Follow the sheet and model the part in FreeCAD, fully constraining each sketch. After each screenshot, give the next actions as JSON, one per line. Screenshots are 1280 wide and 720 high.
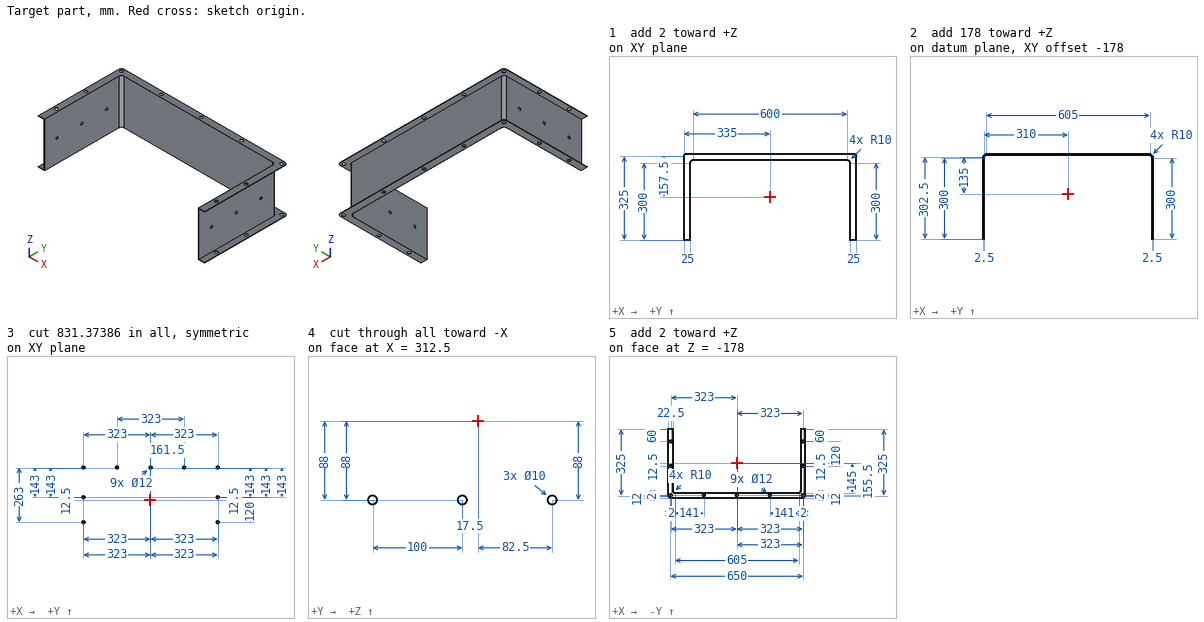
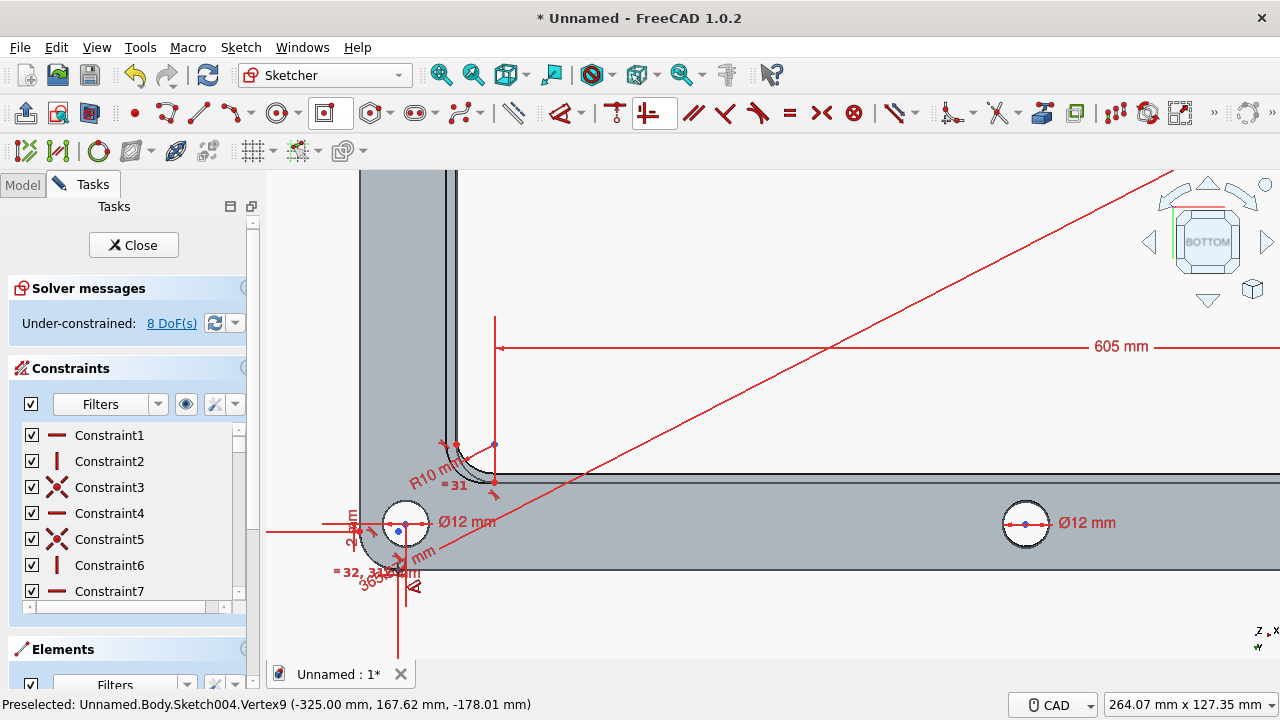
{"action": "left_click", "coordinate": [1026, 525]}
{"action": "left_click", "coordinate": [1060, 548]}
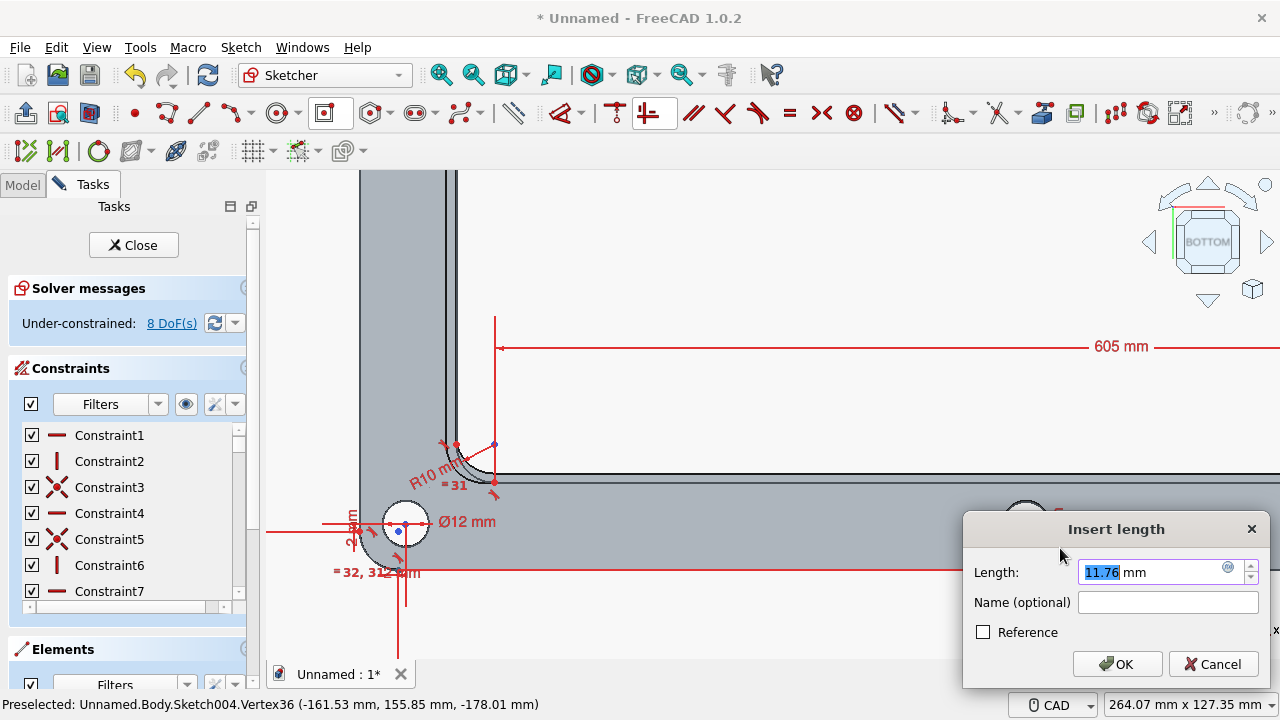
{"action": "type", "text": "12"}
{"action": "key", "text": "Return"}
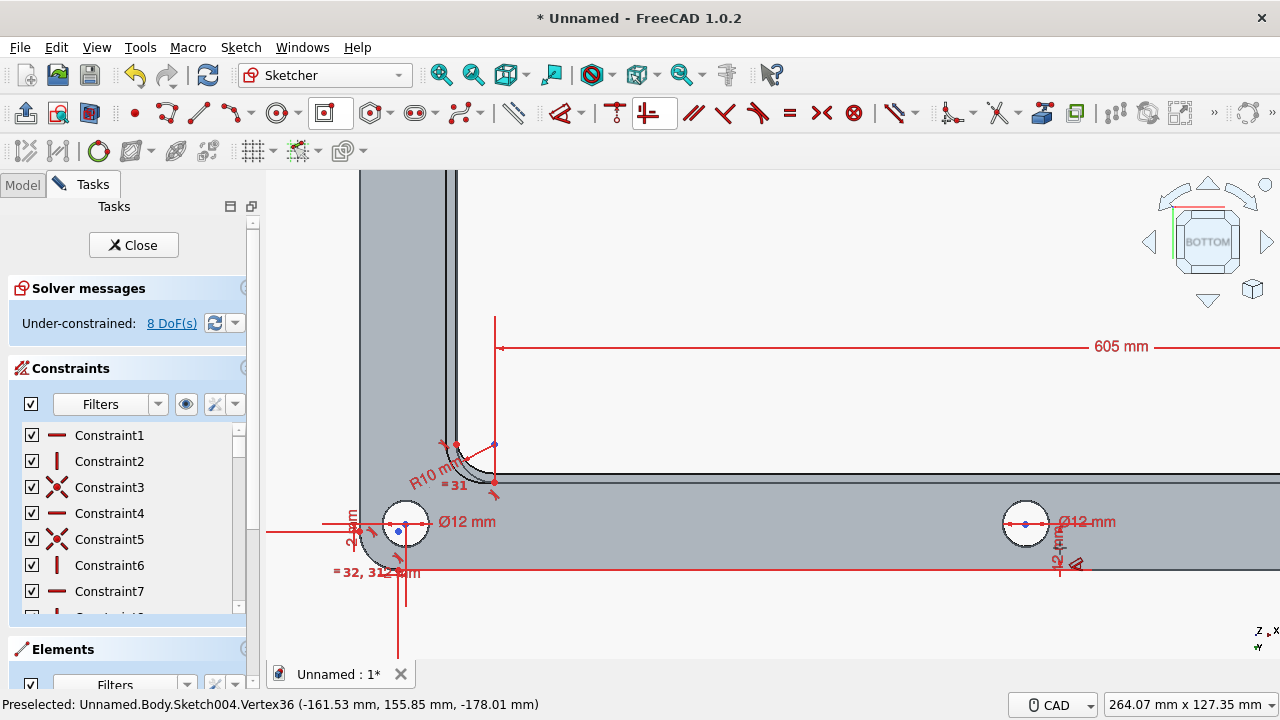
{"action": "scroll", "coordinate": [396, 574], "scroll_direction": "down", "scroll_amount": 7}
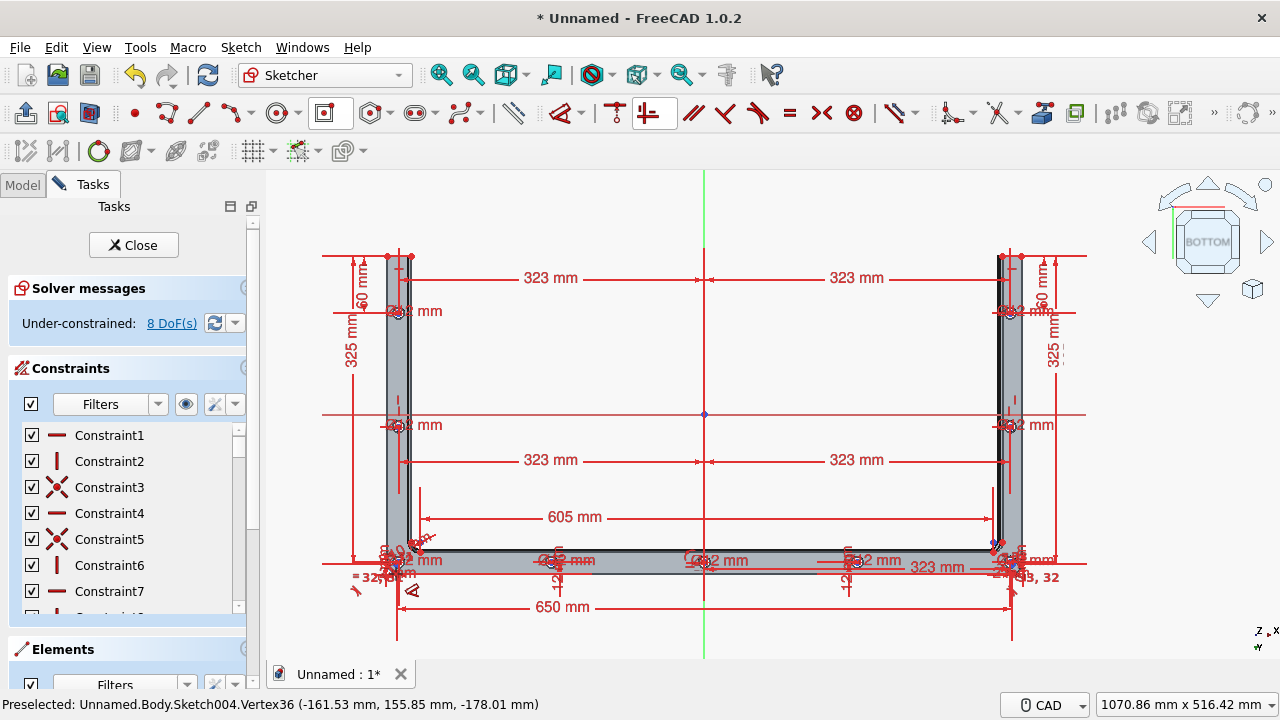
{"action": "scroll", "coordinate": [404, 256], "scroll_direction": "up", "scroll_amount": 4}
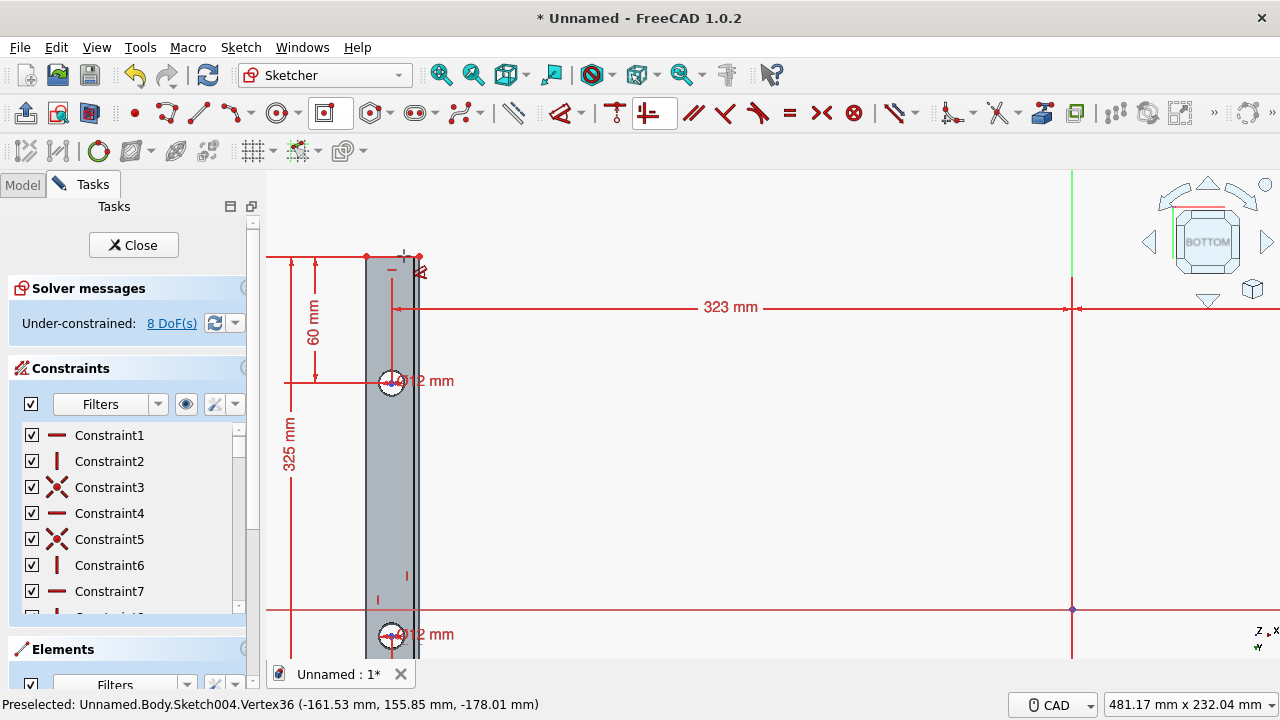
{"action": "left_click", "coordinate": [404, 257]}
{"action": "left_click", "coordinate": [393, 223]}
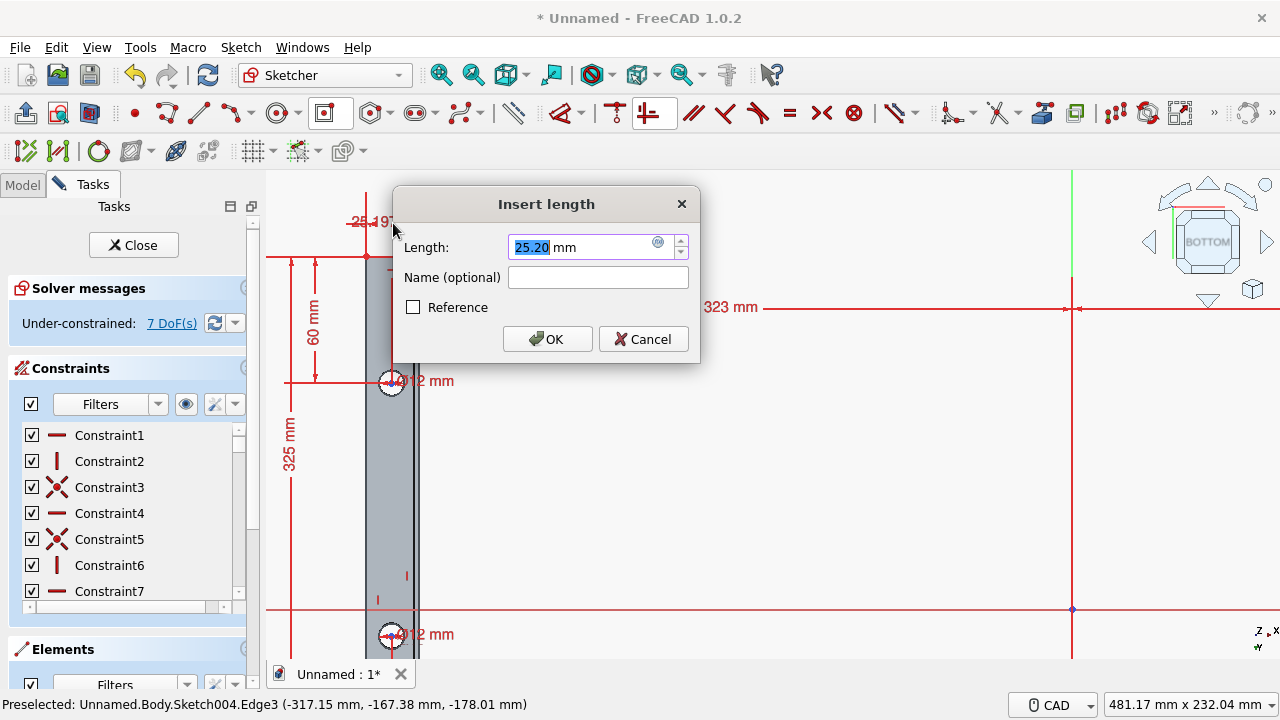
{"action": "type", "text": "22.5"}
{"action": "key", "text": "Return"}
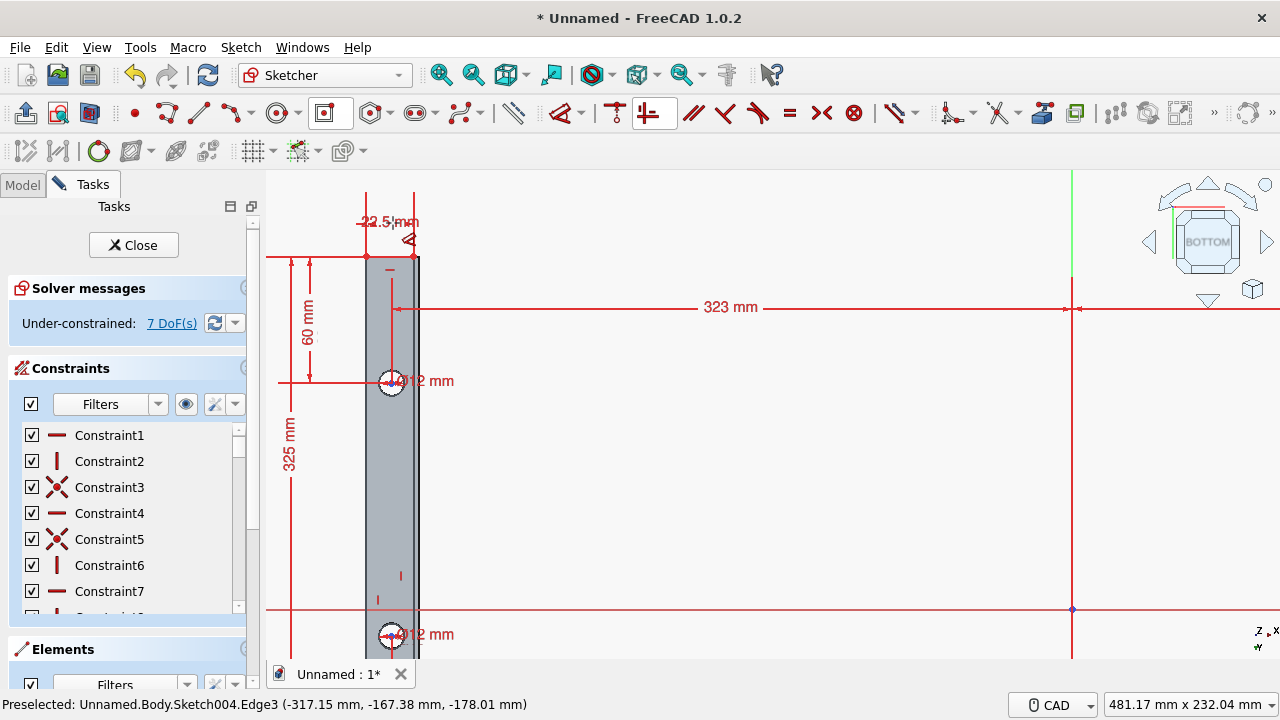
{"action": "scroll", "coordinate": [404, 255], "scroll_direction": "down", "scroll_amount": 4}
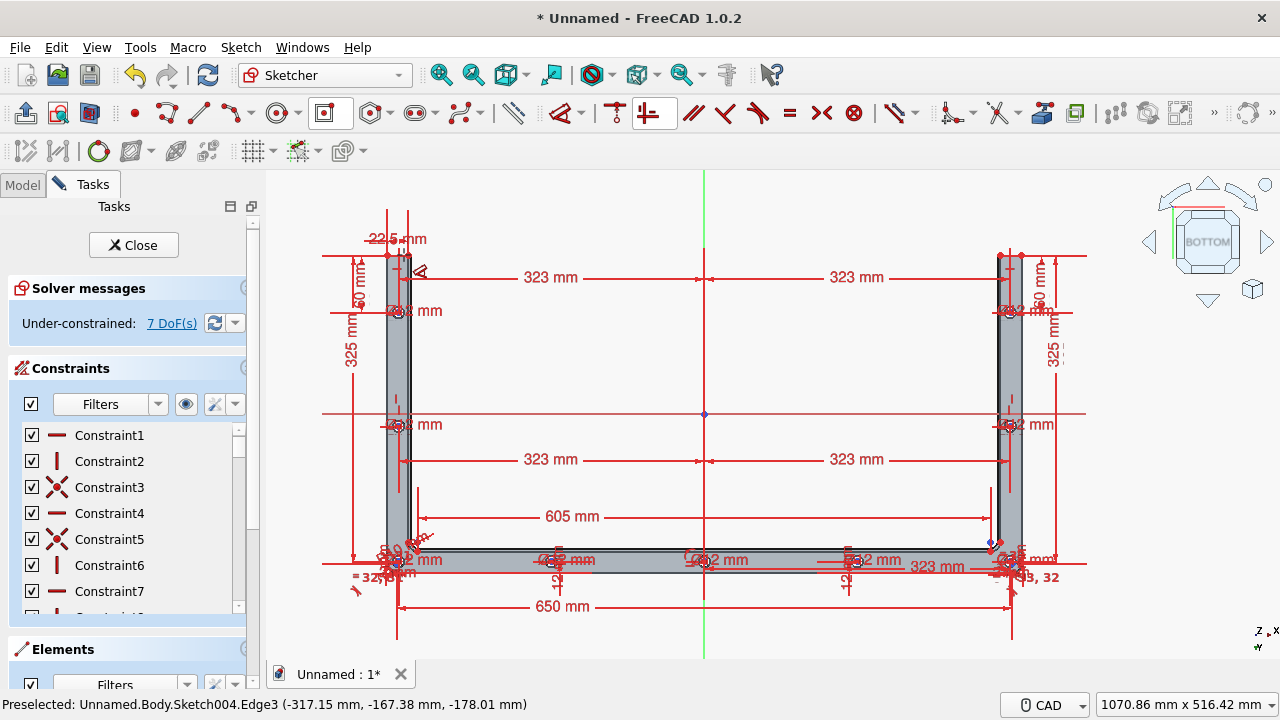
{"action": "scroll", "coordinate": [991, 552], "scroll_direction": "up", "scroll_amount": 2}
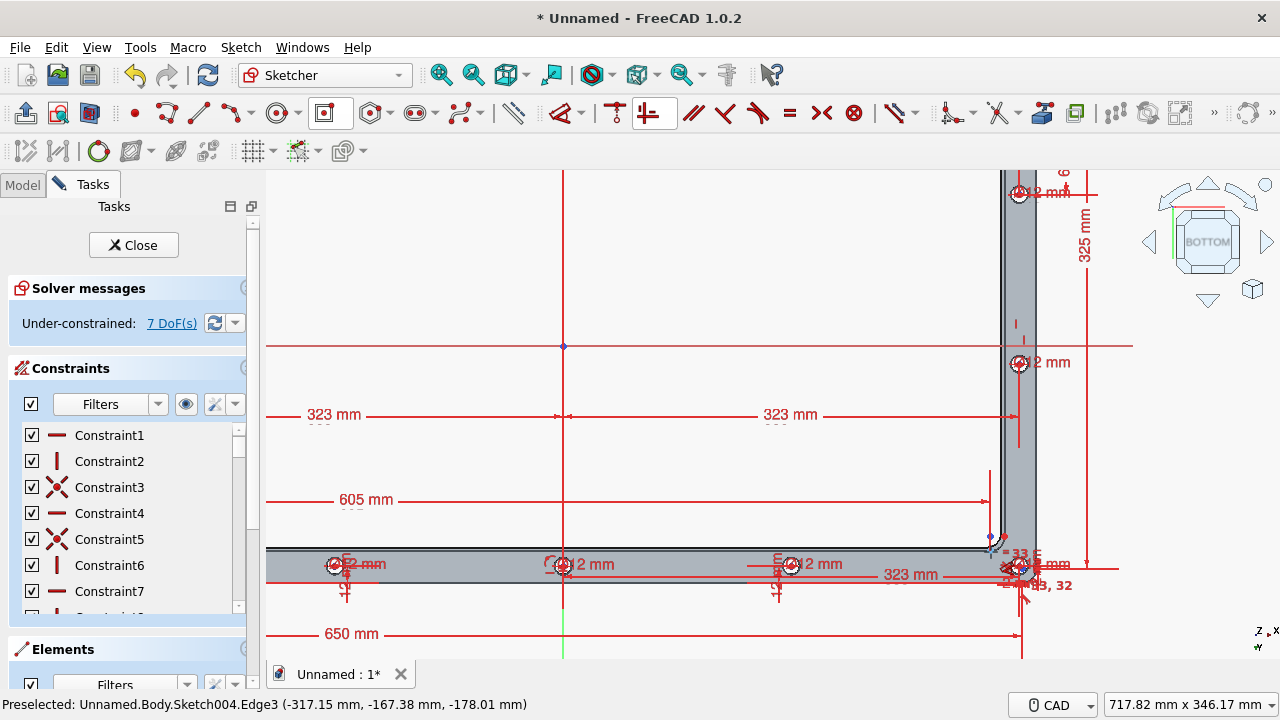
{"action": "left_click", "coordinate": [990, 551]}
{"action": "left_click", "coordinate": [529, 449]}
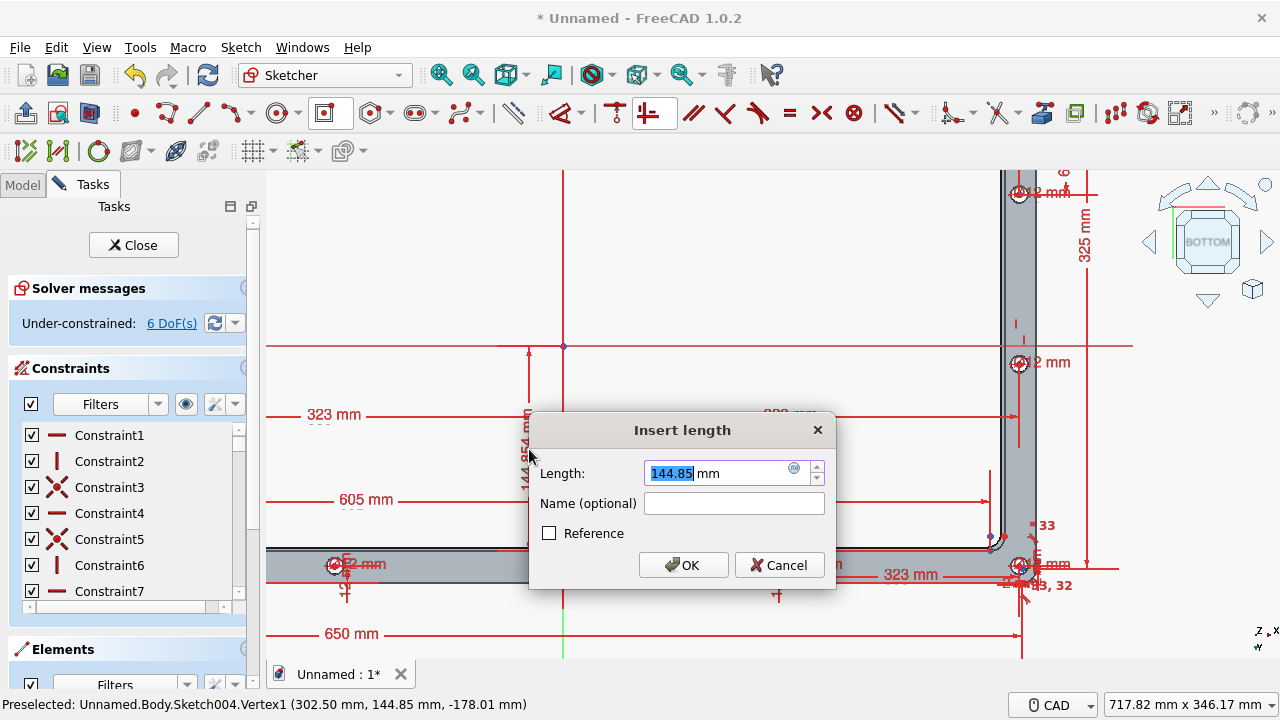
{"action": "type", "text": "145"}
{"action": "key", "text": "Return"}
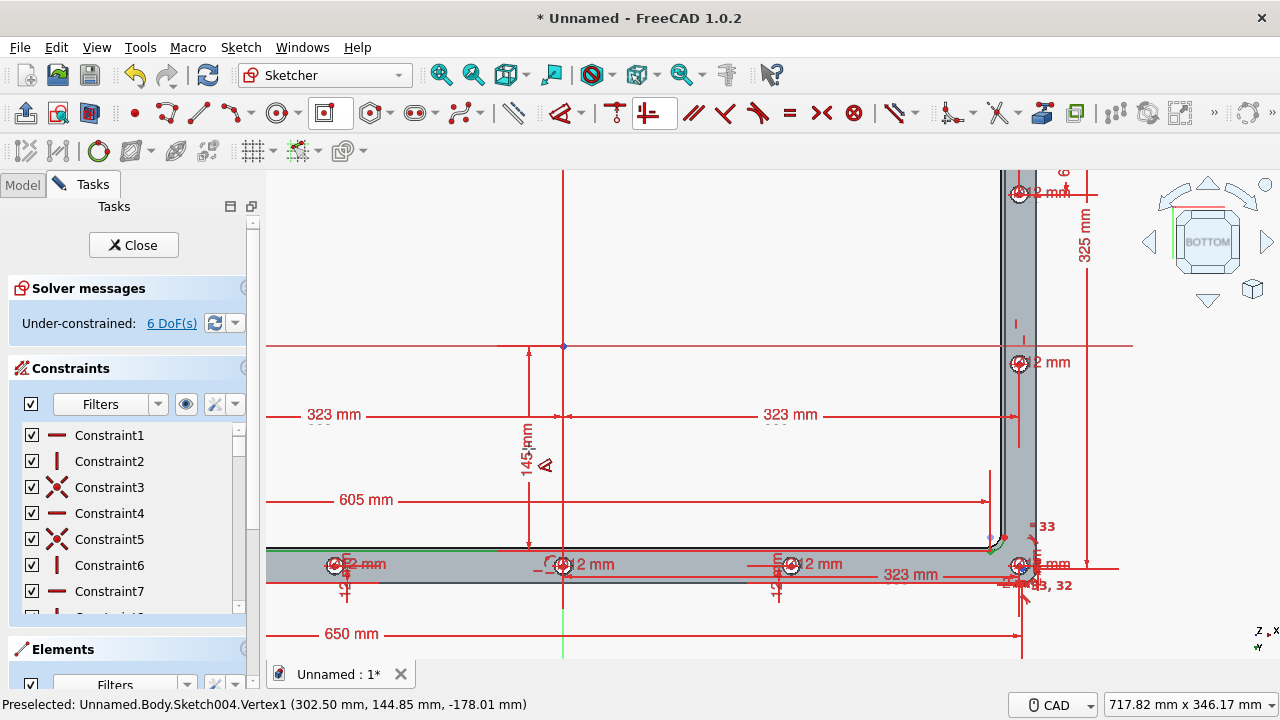
{"action": "scroll", "coordinate": [1019, 364], "scroll_direction": "up", "scroll_amount": 5}